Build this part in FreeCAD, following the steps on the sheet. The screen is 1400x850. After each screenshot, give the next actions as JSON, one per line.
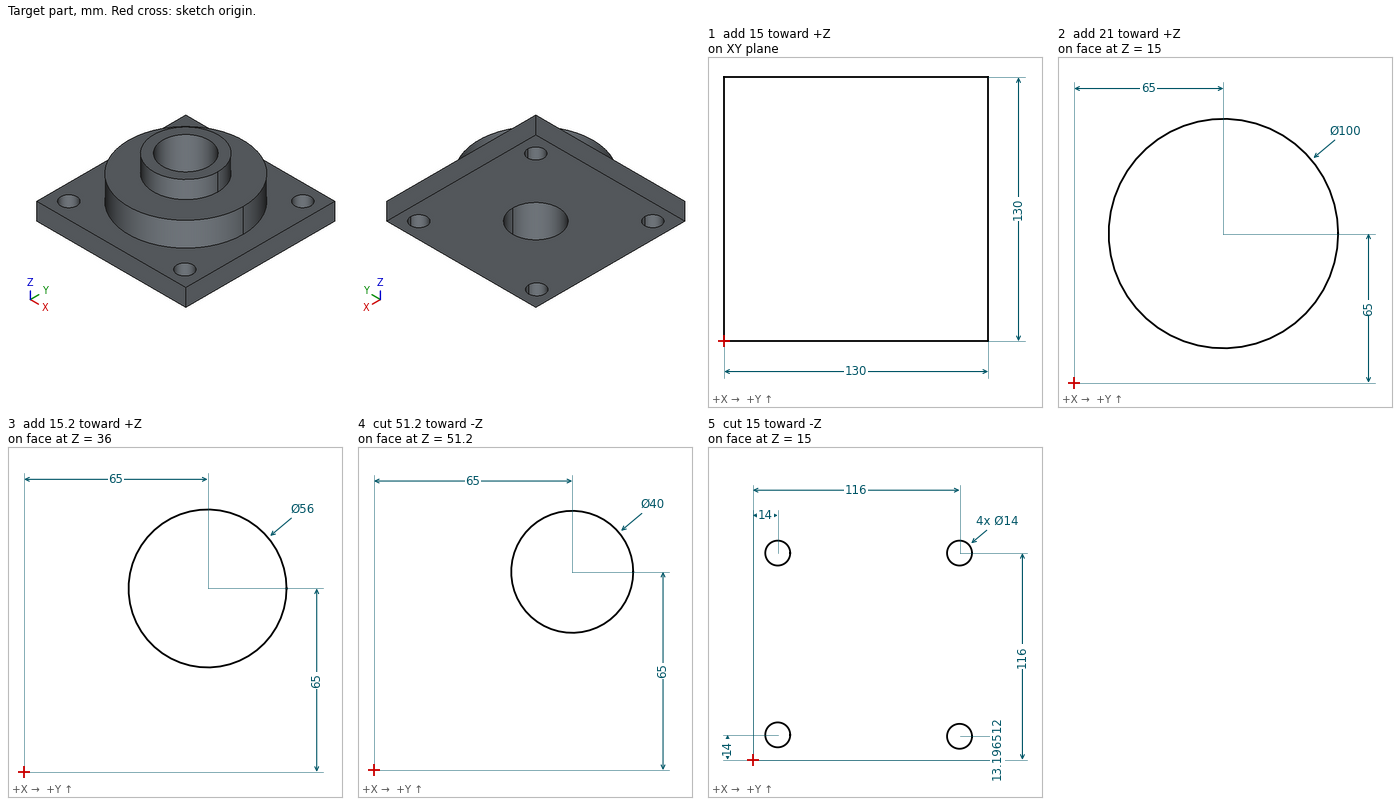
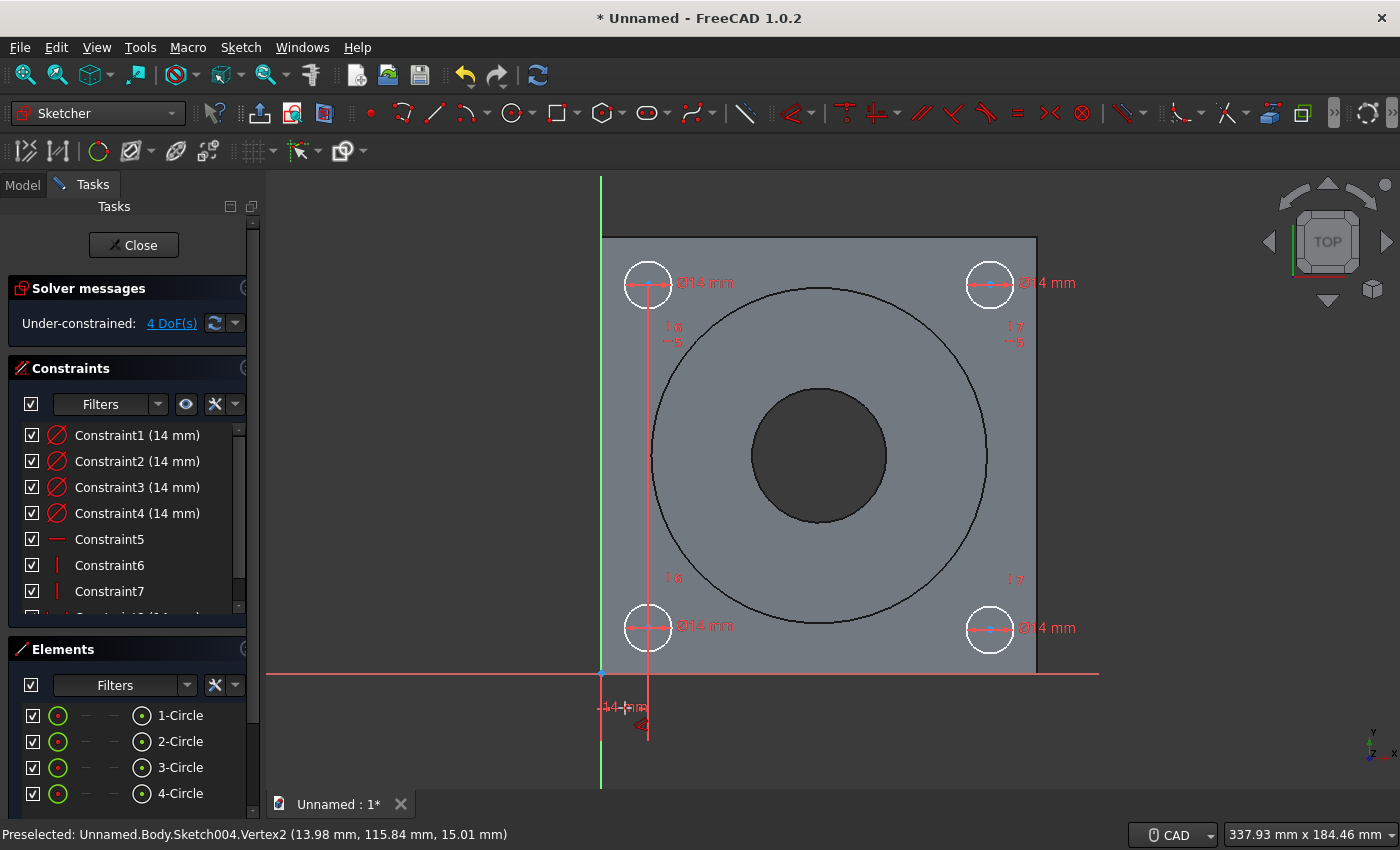
{"action": "left_click", "coordinate": [648, 628]}
{"action": "left_click", "coordinate": [567, 651]}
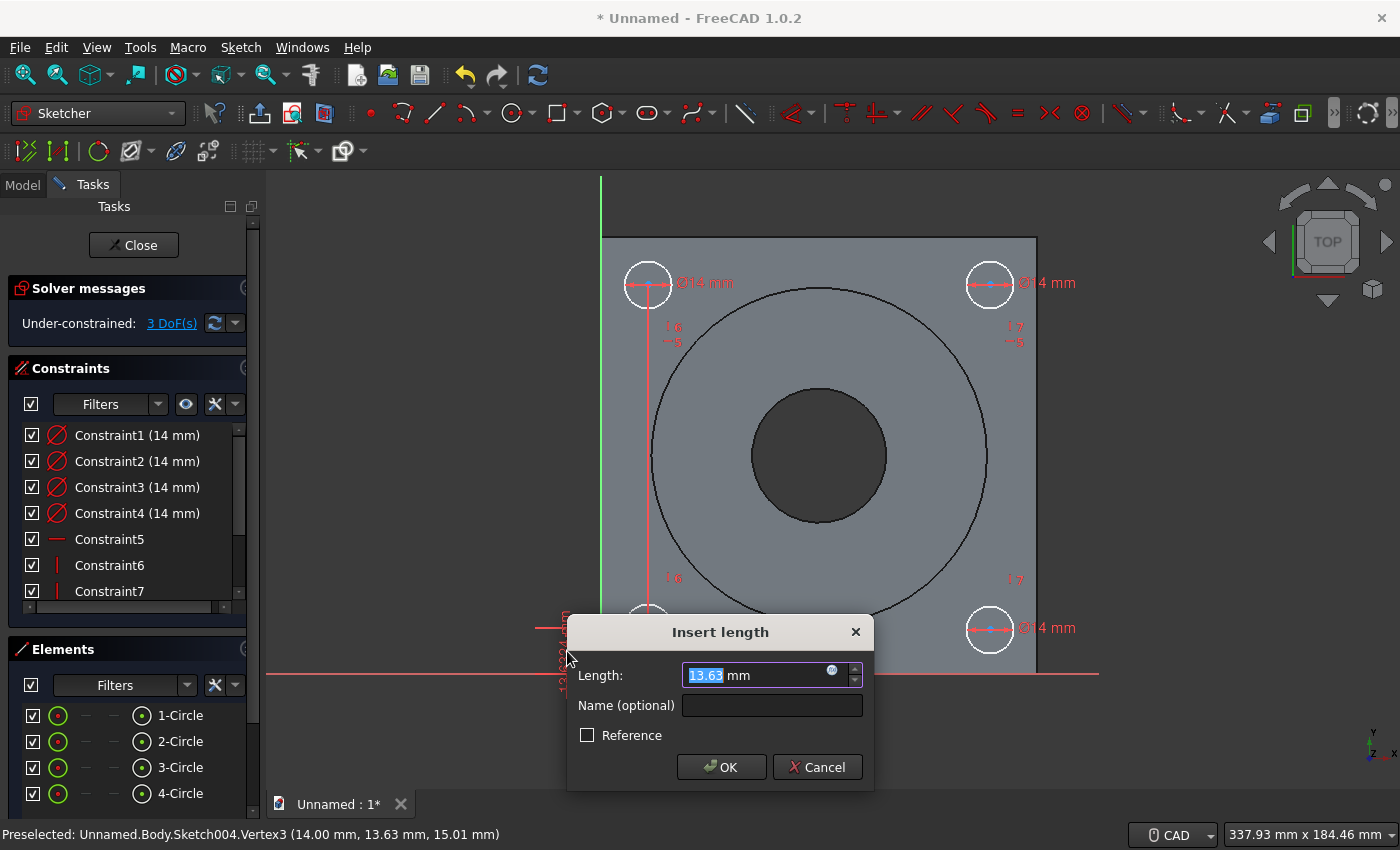
{"action": "type", "text": "14"}
{"action": "key", "text": "Return"}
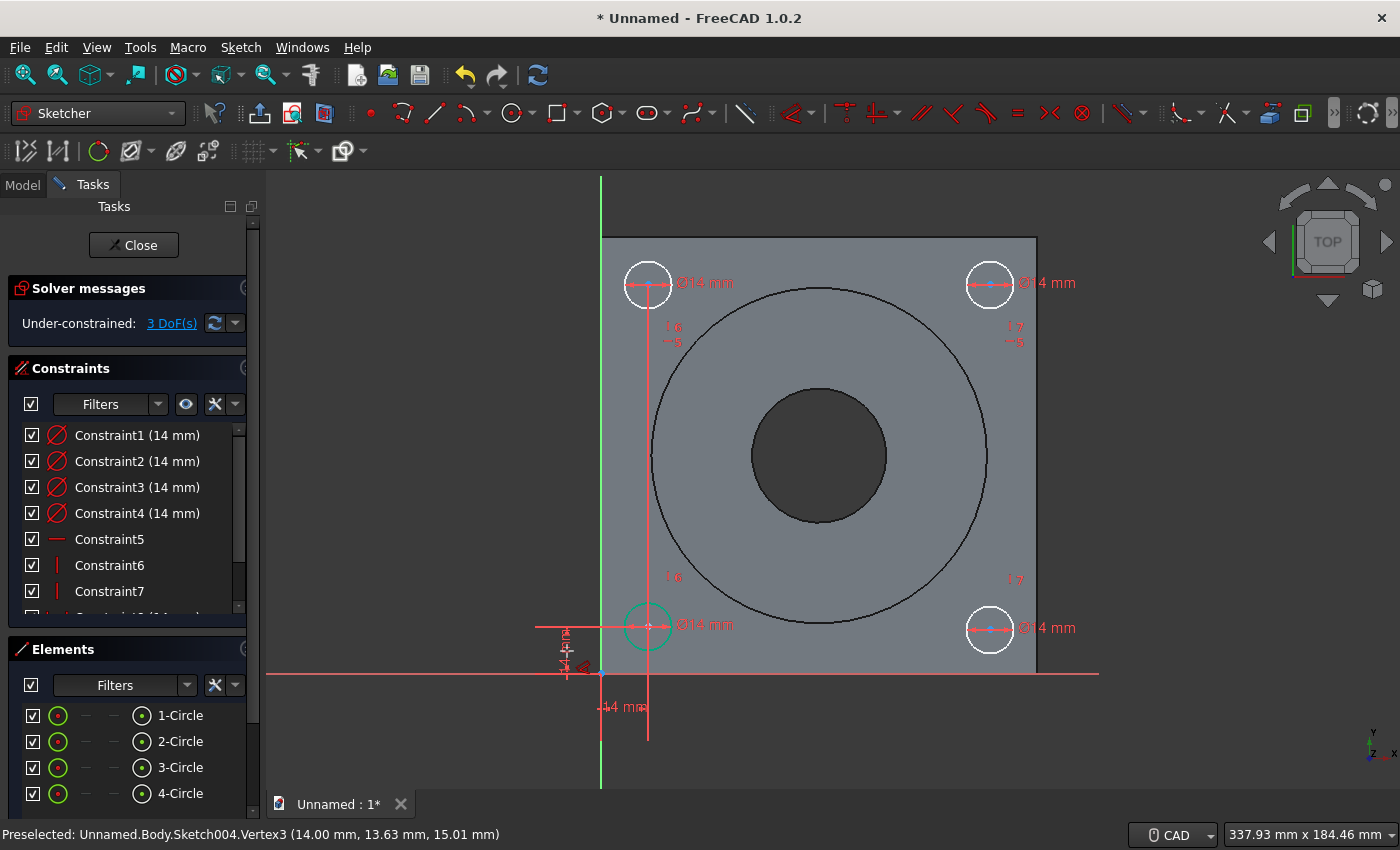
{"action": "left_click", "coordinate": [990, 285]}
{"action": "left_click", "coordinate": [796, 708]}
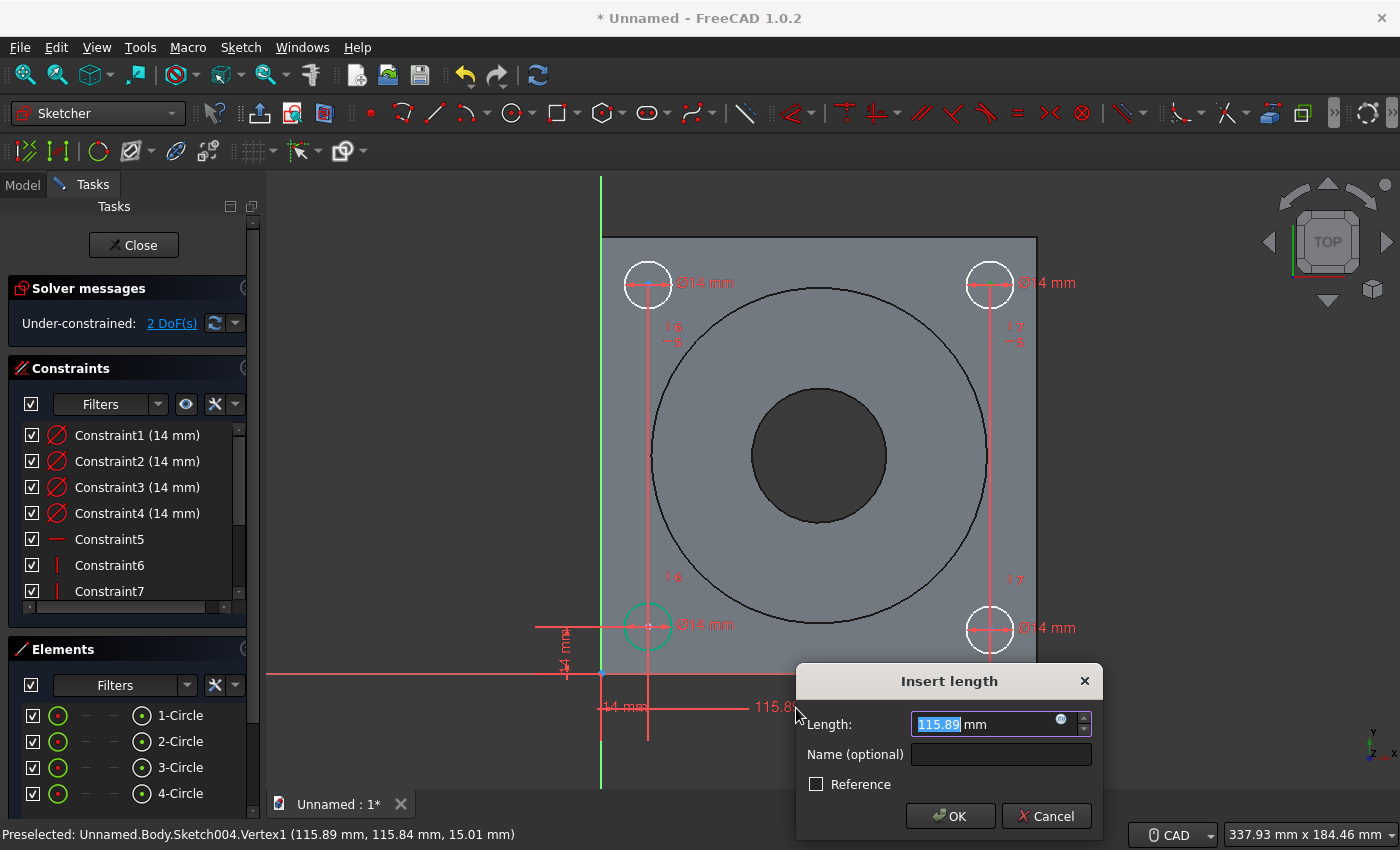
{"action": "type", "text": "116"}
{"action": "key", "text": "Return"}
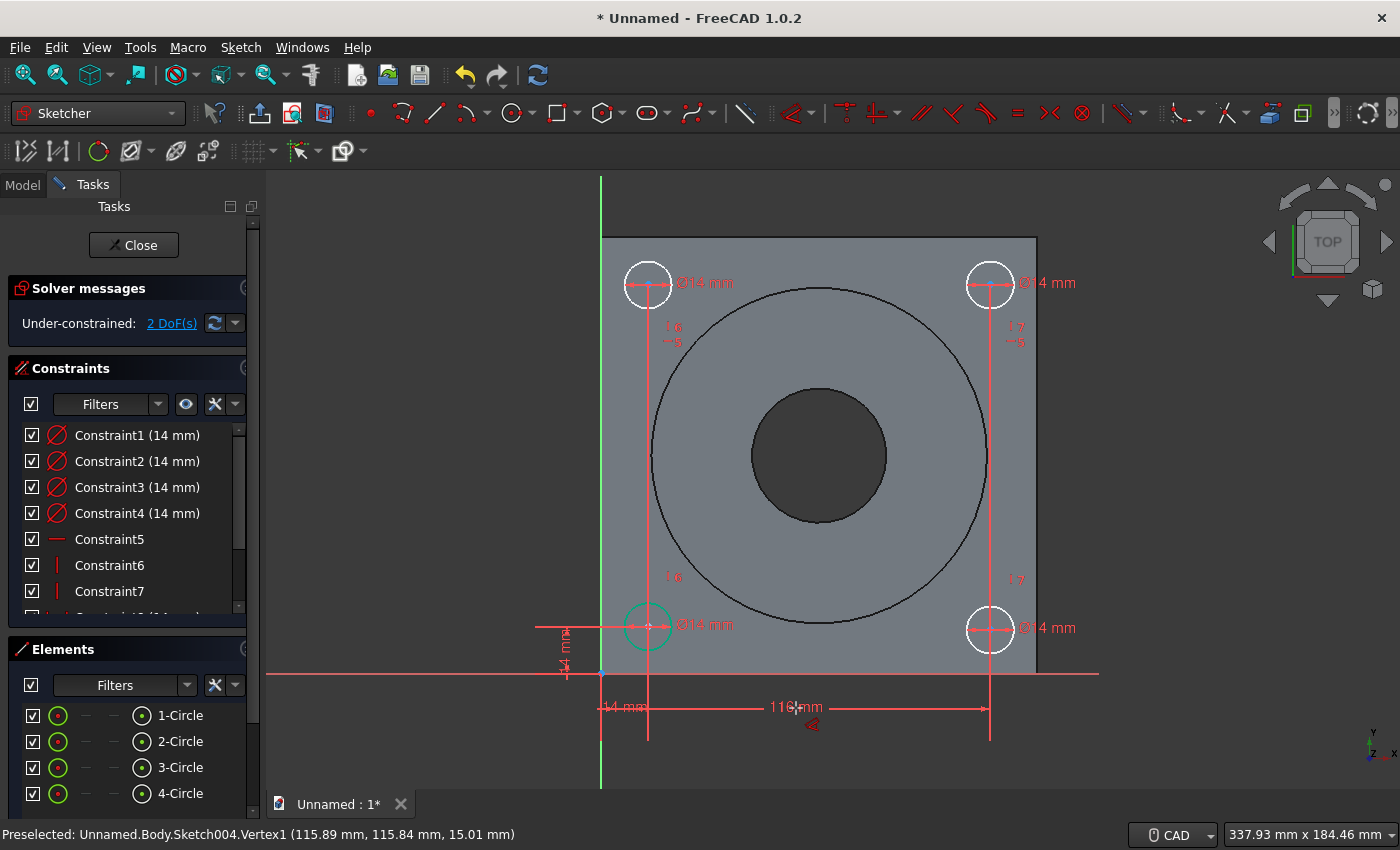
{"action": "left_click", "coordinate": [990, 285]}
{"action": "left_click", "coordinate": [567, 479]}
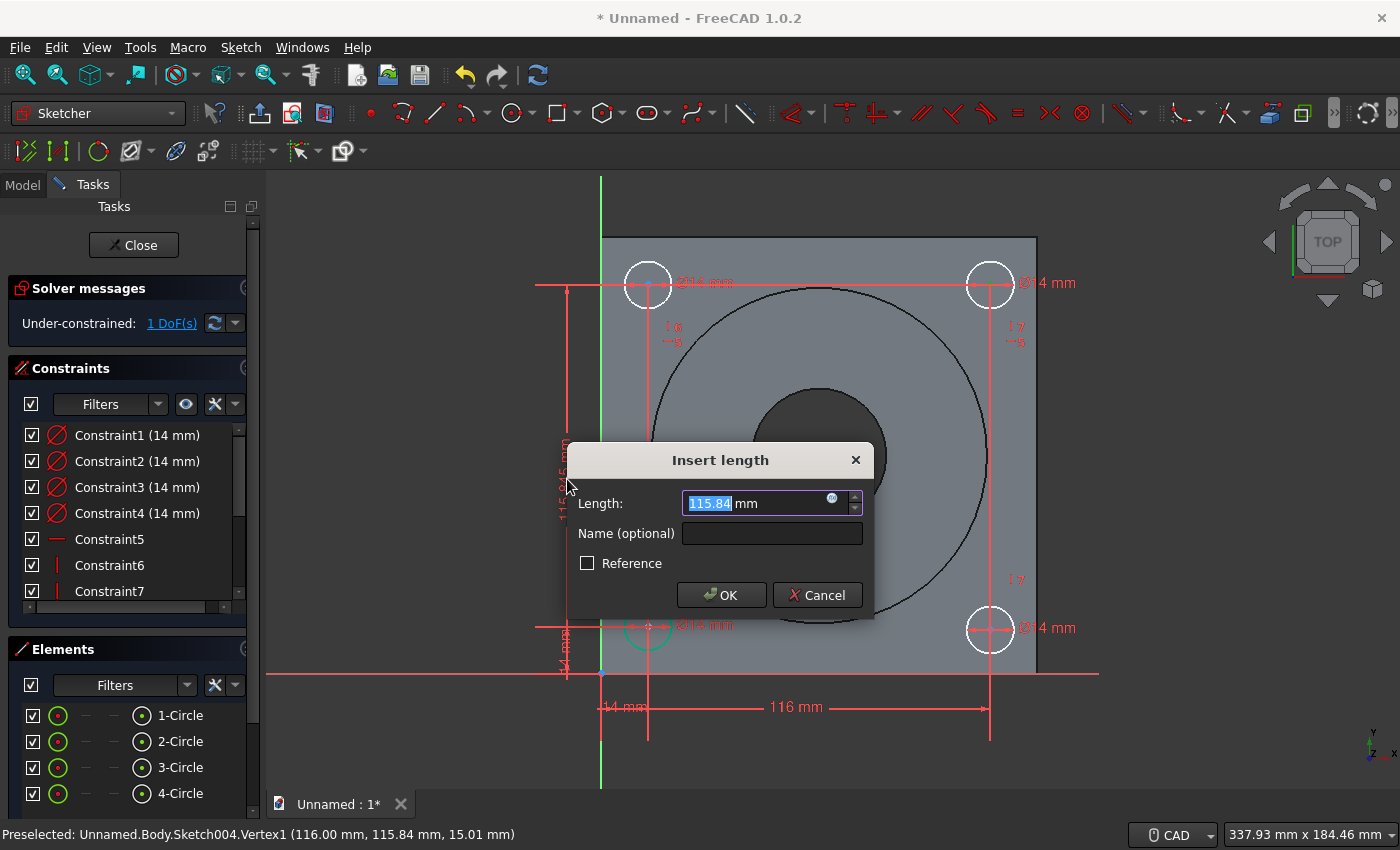
{"action": "type", "text": "116"}
{"action": "key", "text": "Return"}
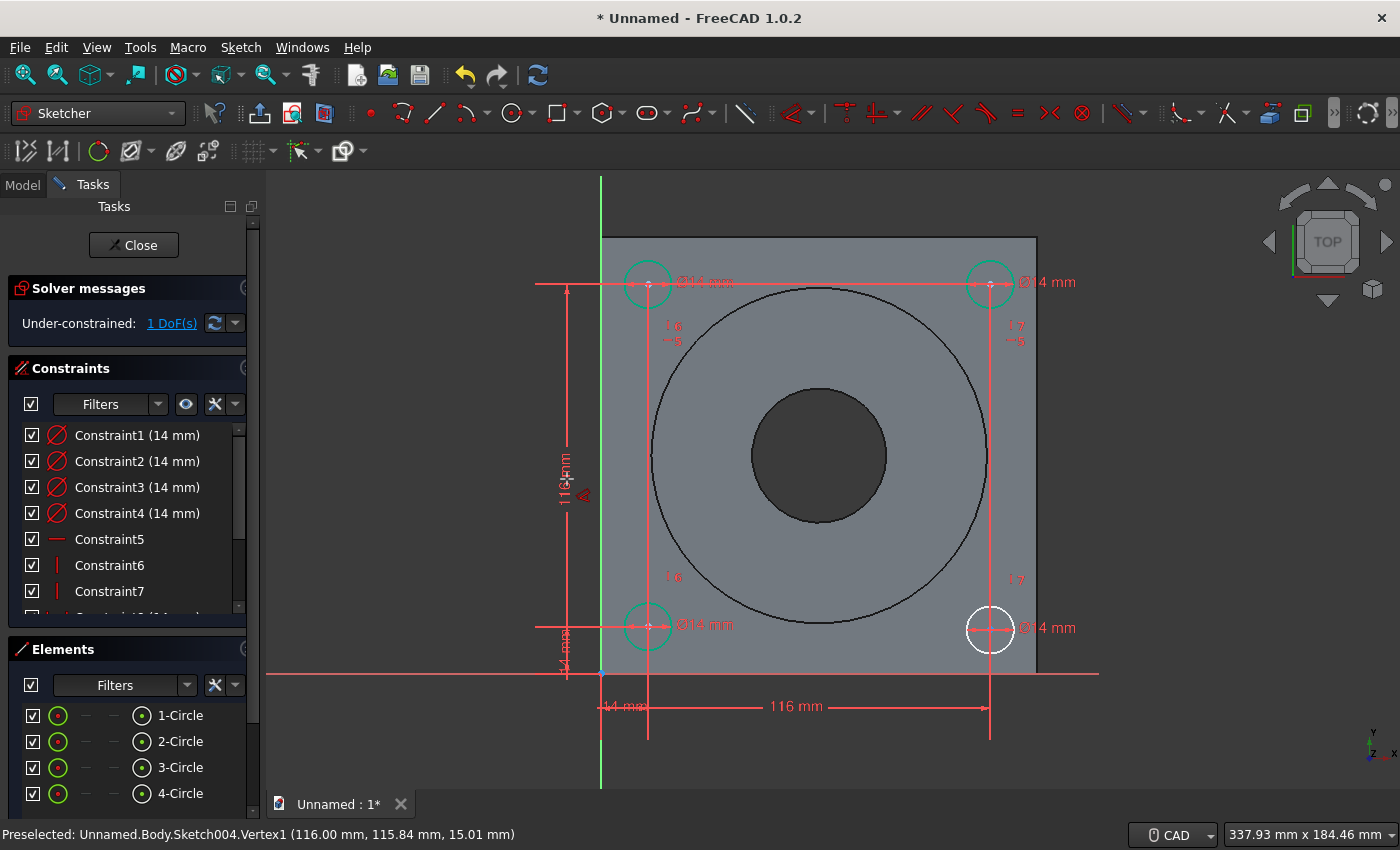
{"action": "left_click", "coordinate": [990, 630]}
{"action": "left_click", "coordinate": [1024, 652]}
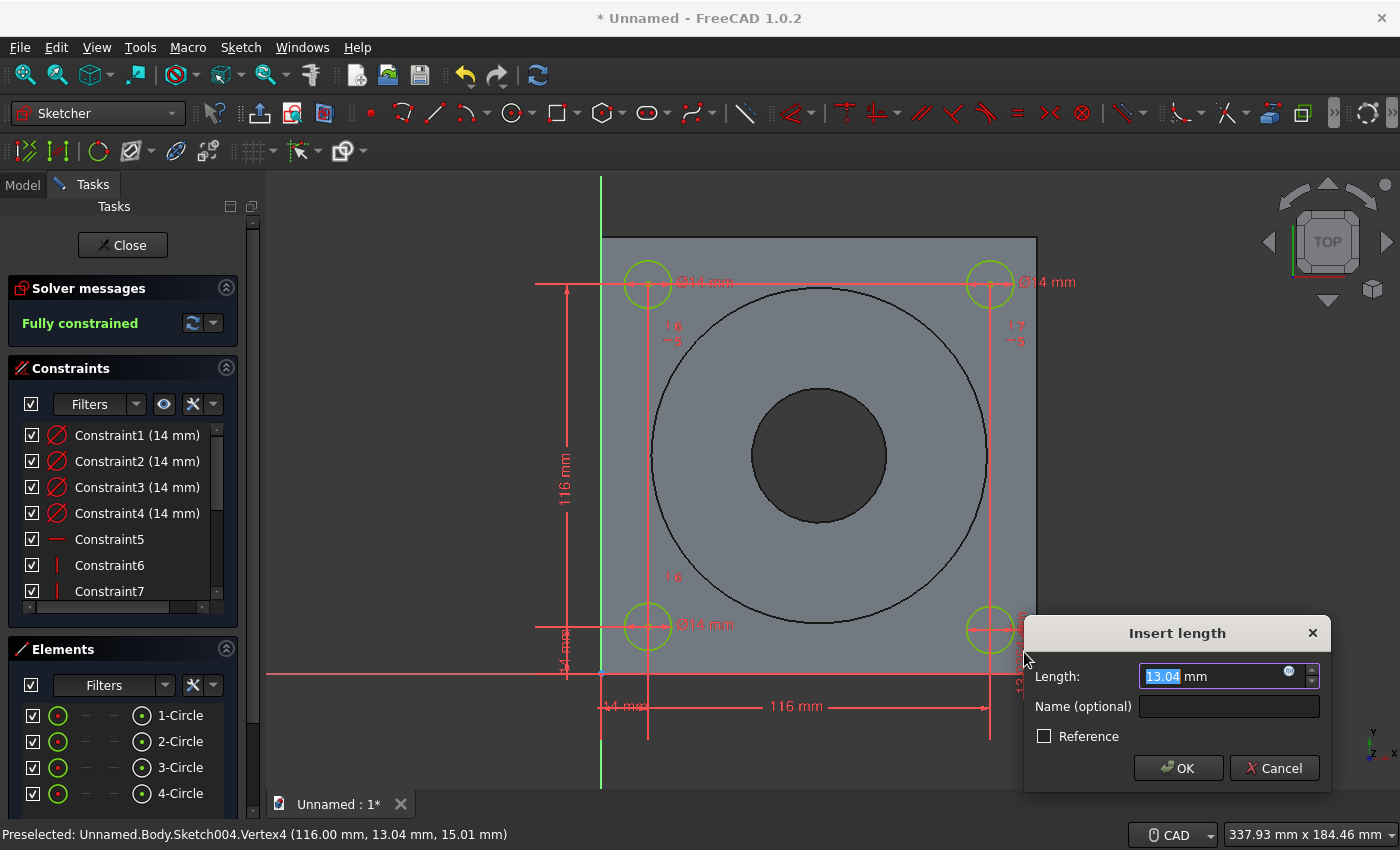
{"action": "type", "text": "13.196512"}
{"action": "key", "text": "Return"}
{"action": "key", "text": "Escape"}